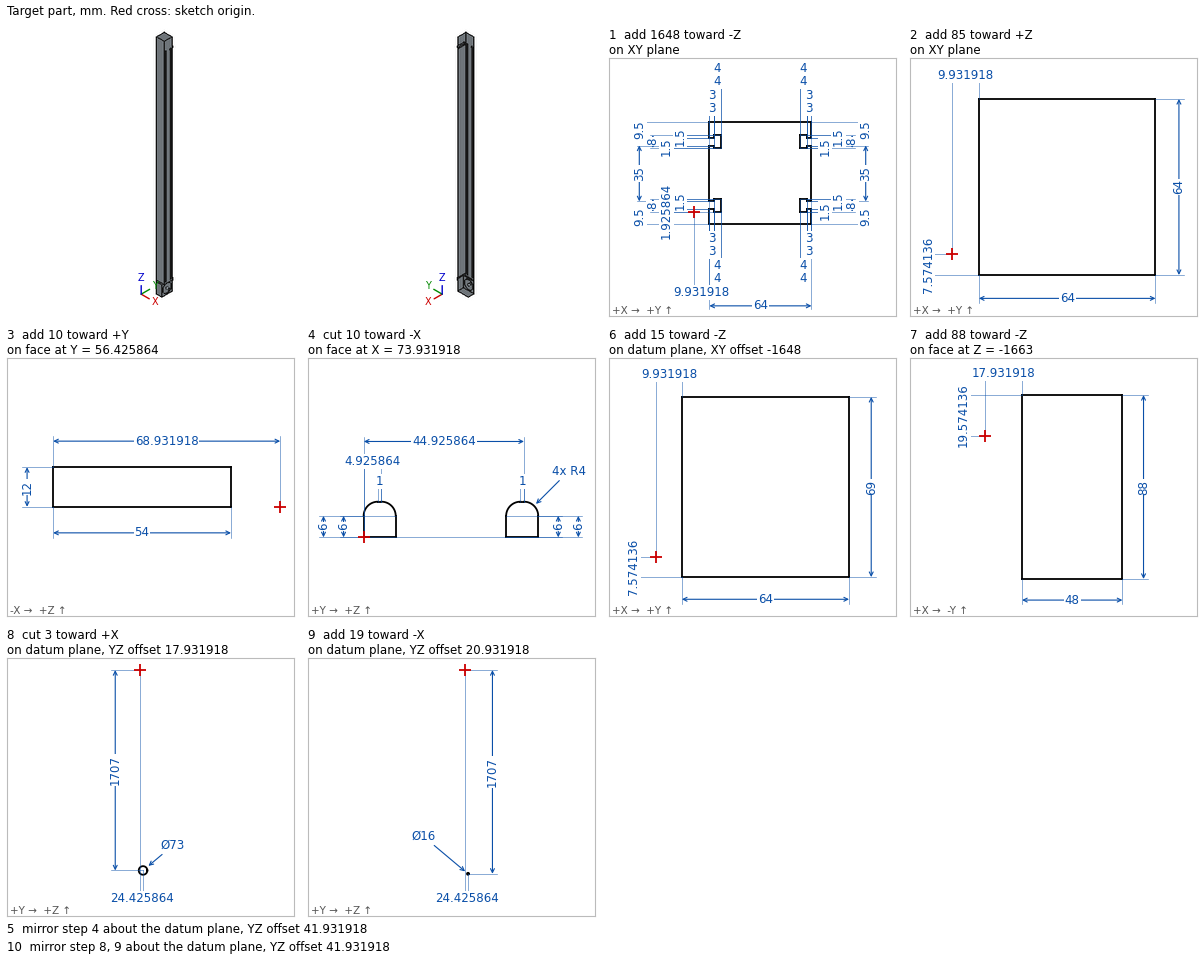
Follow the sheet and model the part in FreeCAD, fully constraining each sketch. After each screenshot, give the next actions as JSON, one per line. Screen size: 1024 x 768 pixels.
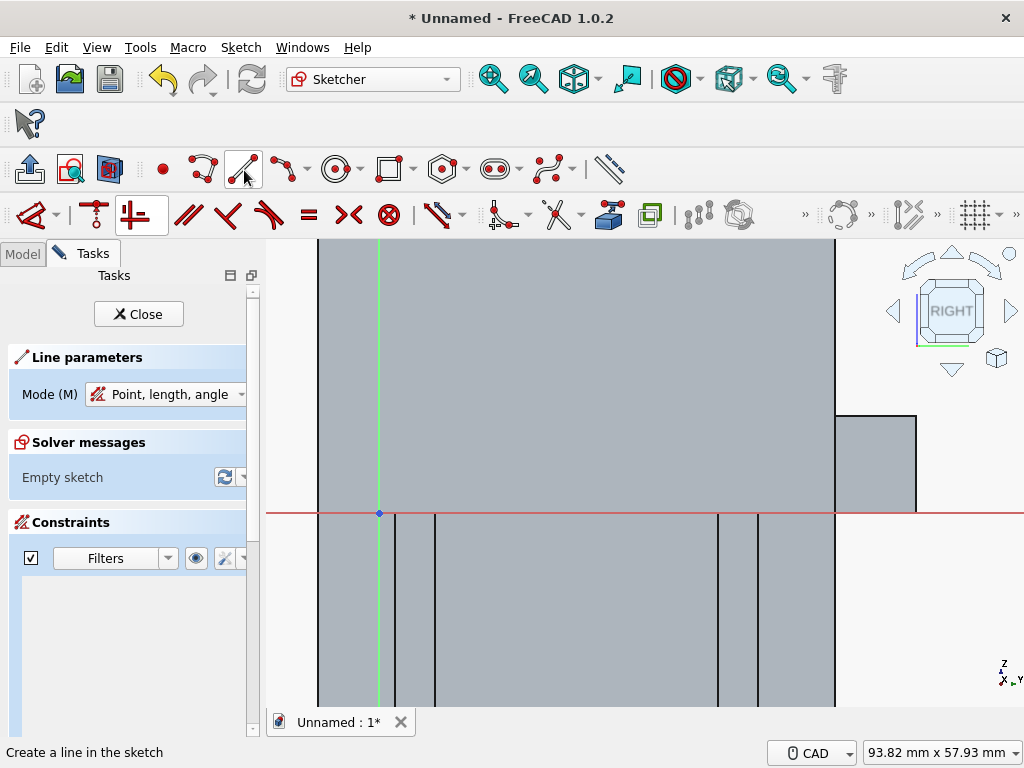
{"action": "left_click", "coordinate": [742, 432]}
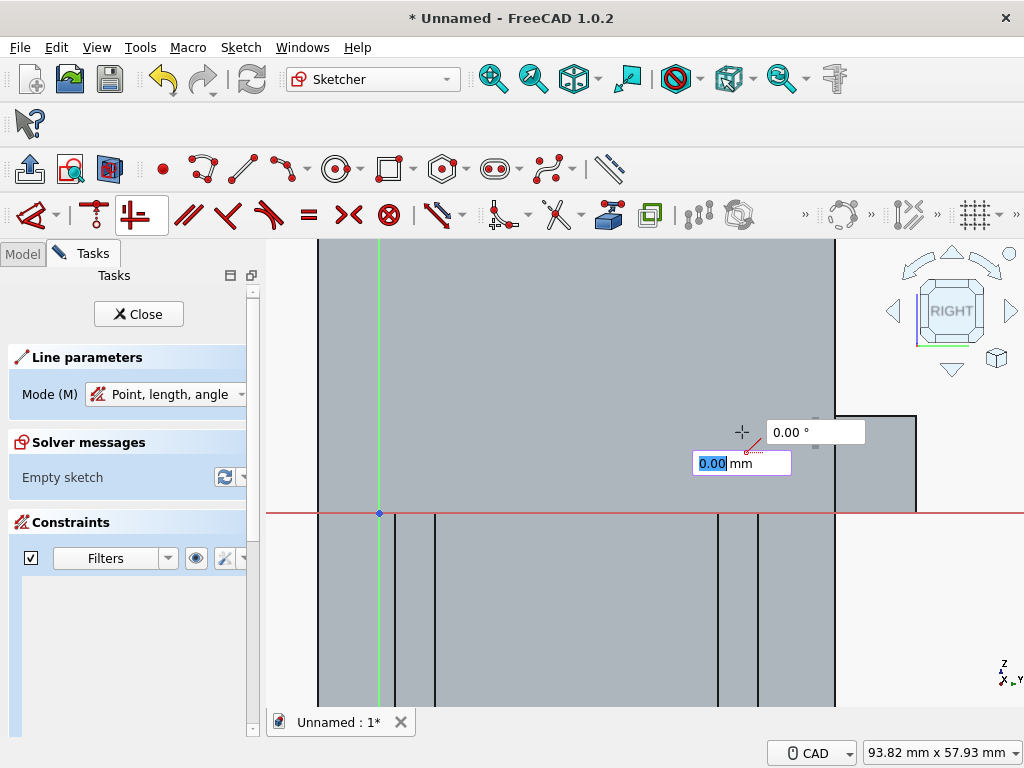
{"action": "scroll", "coordinate": [734, 432], "scroll_direction": "up", "scroll_amount": 4}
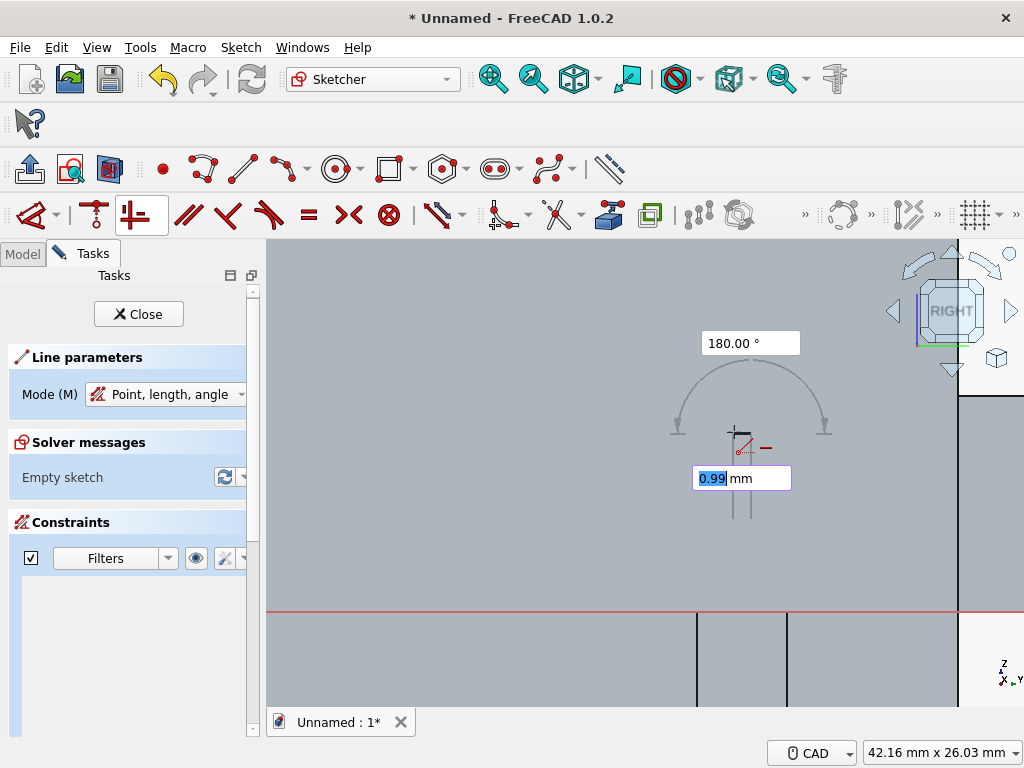
{"action": "left_click", "coordinate": [733, 431]}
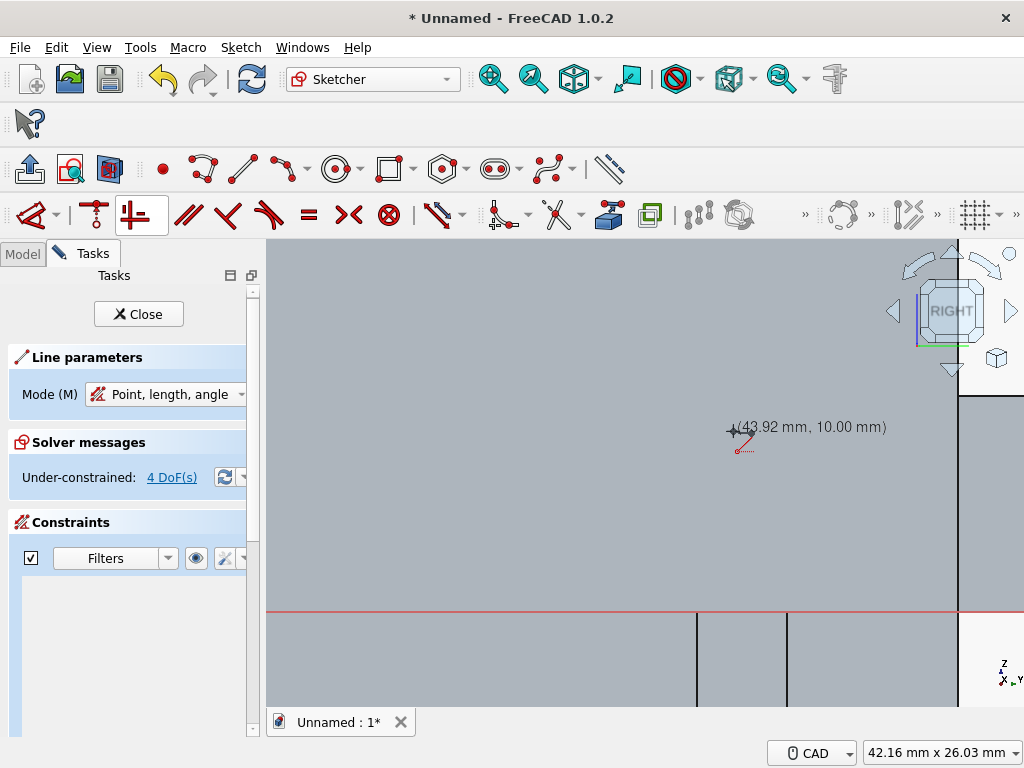
{"action": "left_click", "coordinate": [204, 170]}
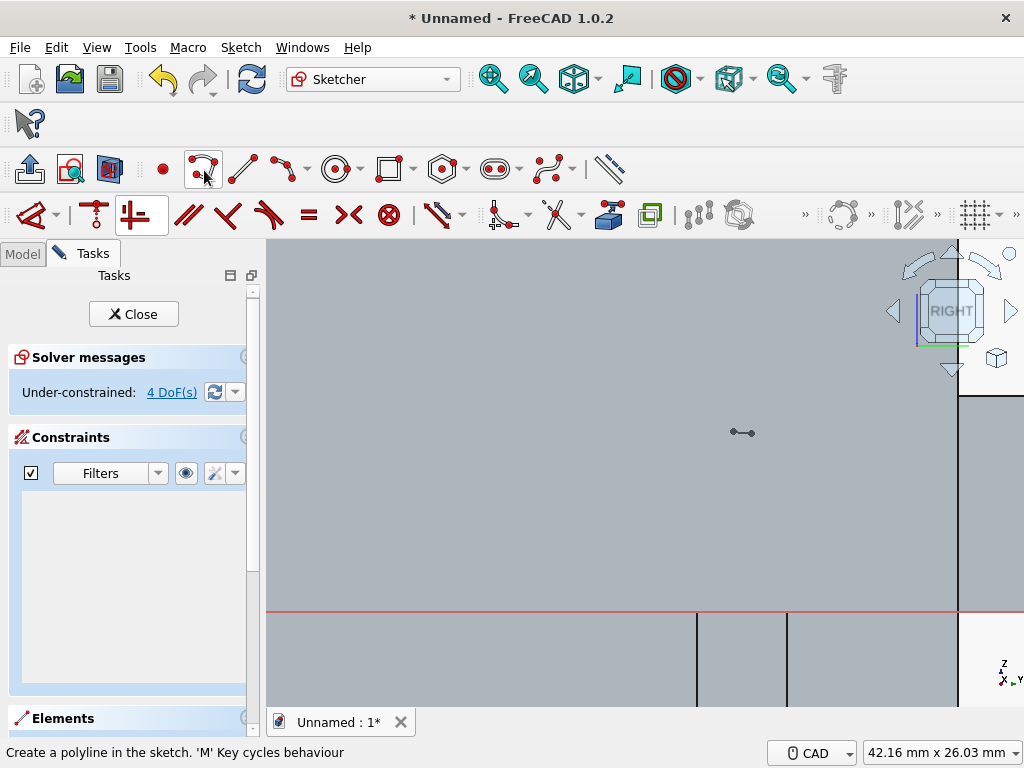
{"action": "left_click", "coordinate": [661, 504]}
{"action": "left_click", "coordinate": [661, 612]}
{"action": "left_click", "coordinate": [823, 603]}
{"action": "left_click", "coordinate": [823, 504]}
{"action": "right_click", "coordinate": [823, 504]}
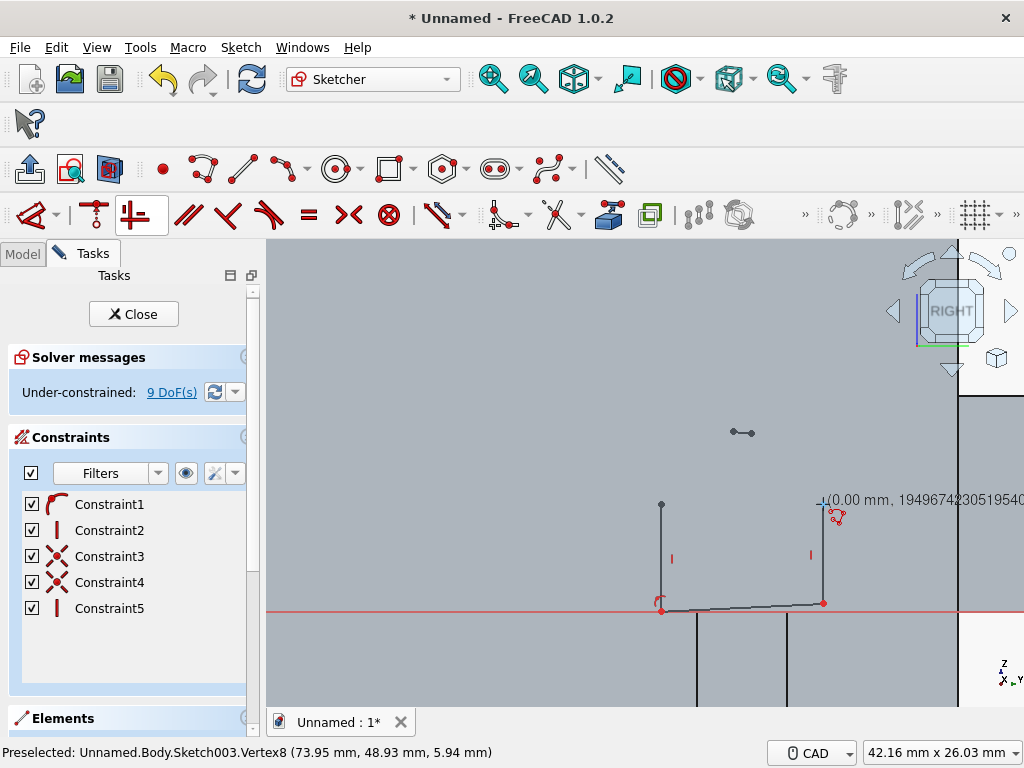
{"action": "left_click", "coordinate": [284, 170]}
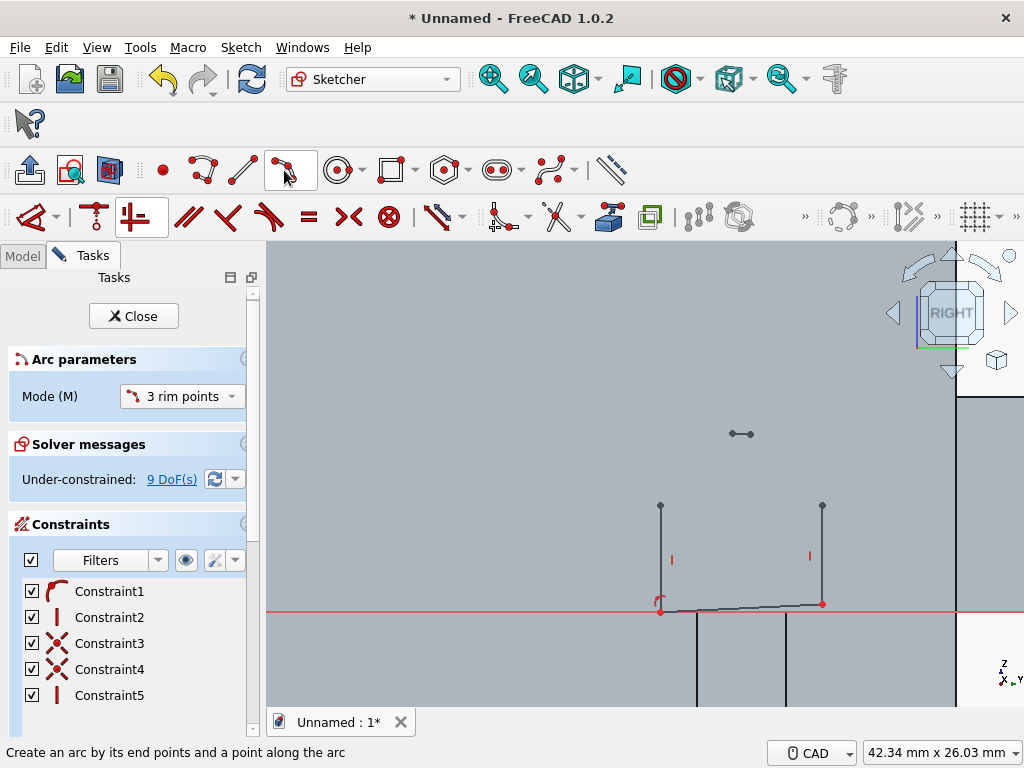
{"action": "scroll", "coordinate": [733, 433], "scroll_direction": "up", "scroll_amount": 3}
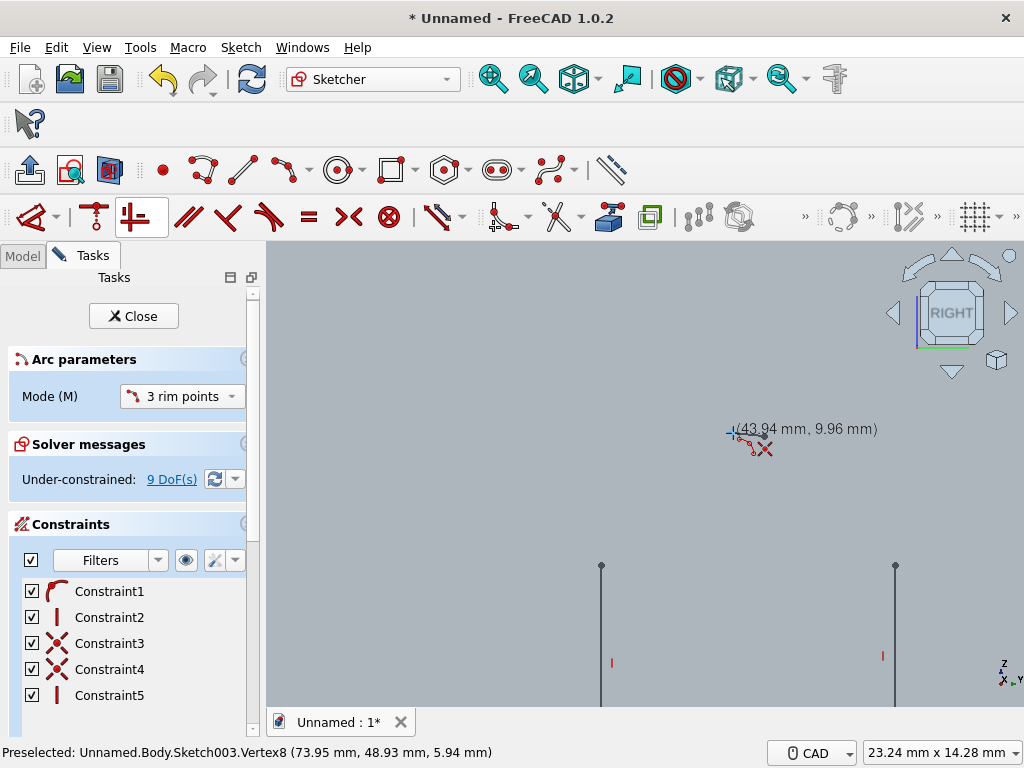
{"action": "left_click", "coordinate": [732, 433]}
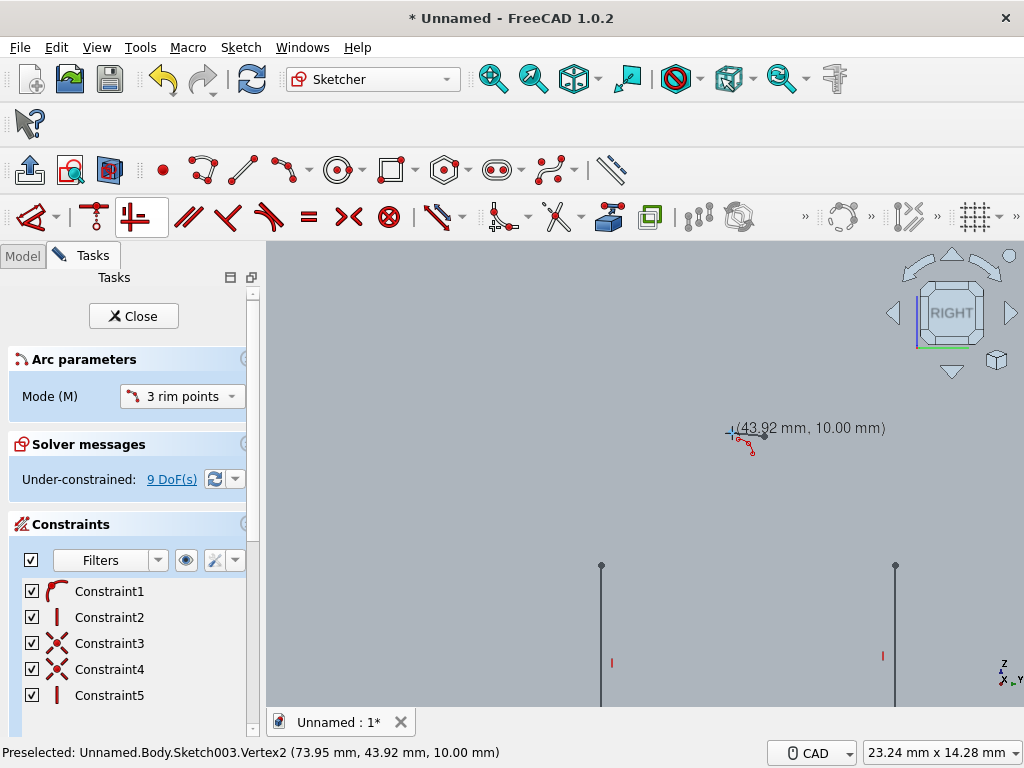
{"action": "scroll", "coordinate": [734, 434], "scroll_direction": "down", "scroll_amount": 7}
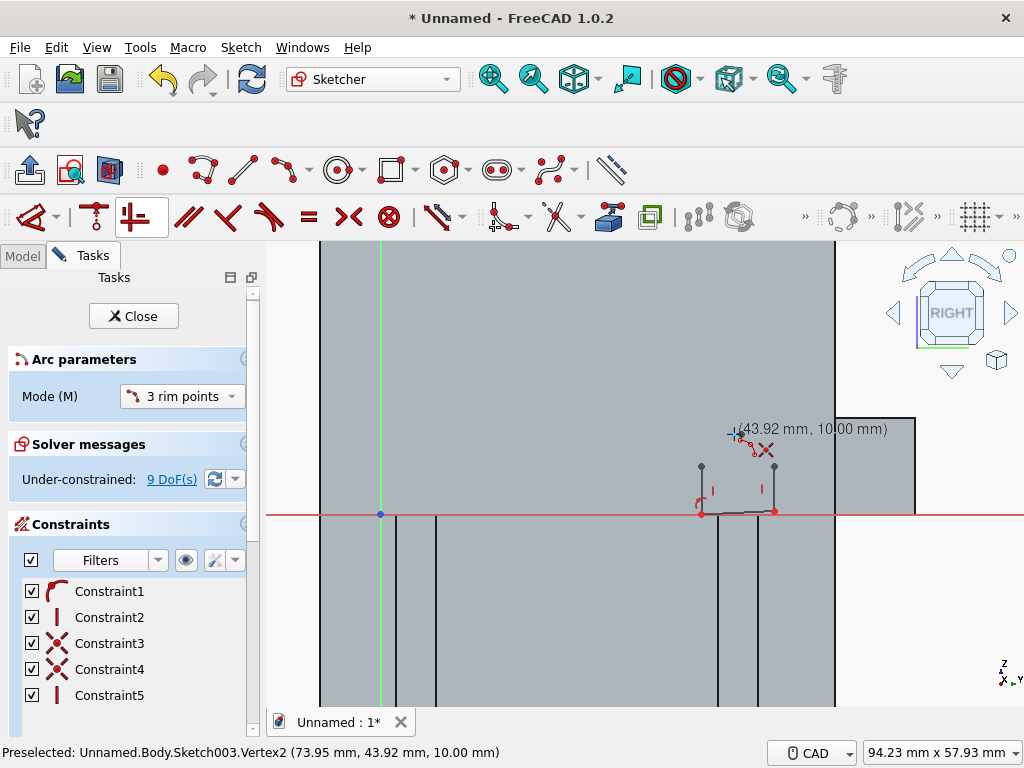
{"action": "left_click", "coordinate": [702, 467]}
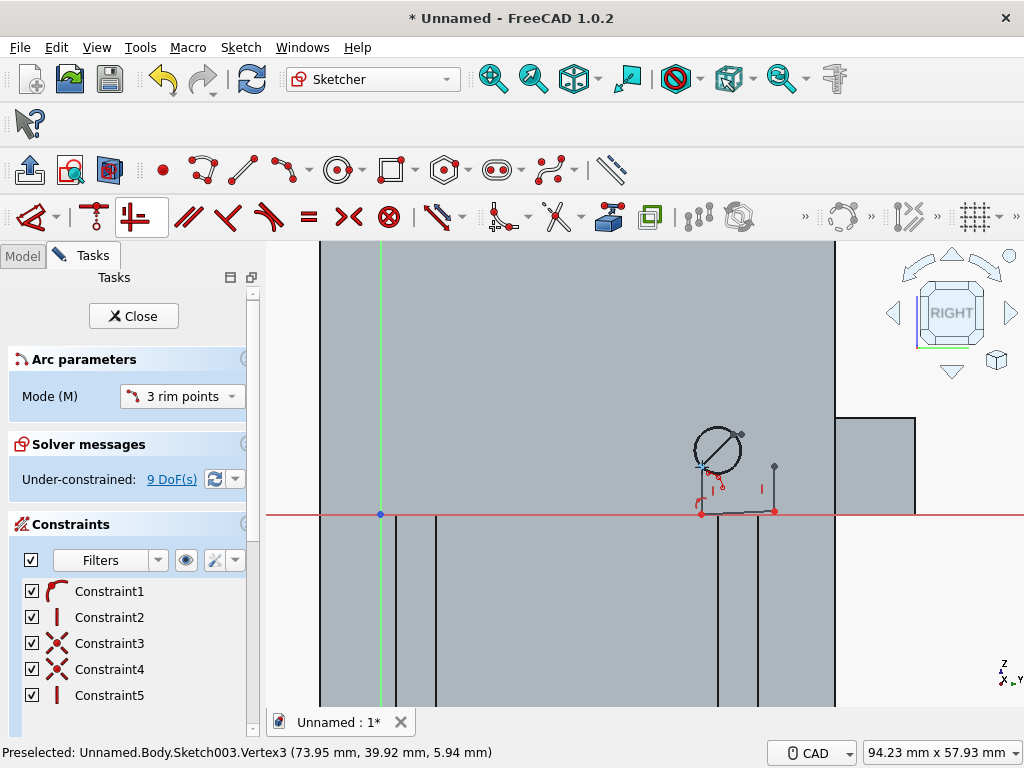
{"action": "scroll", "coordinate": [711, 444], "scroll_direction": "up", "scroll_amount": 3}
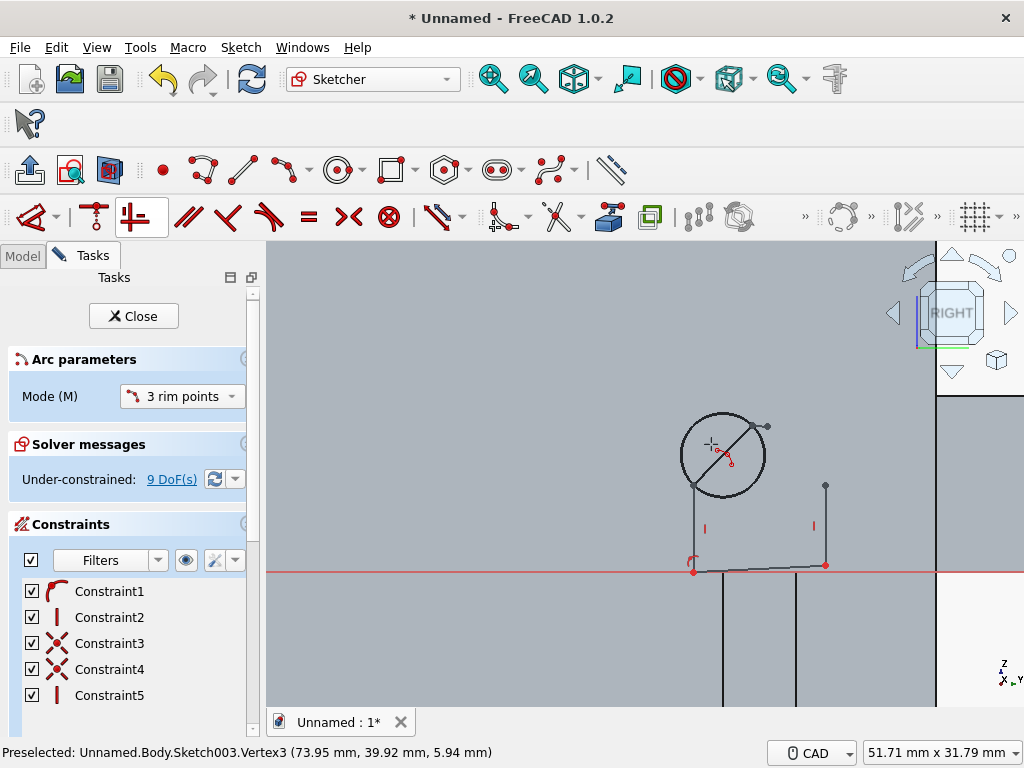
{"action": "left_click", "coordinate": [711, 443]}